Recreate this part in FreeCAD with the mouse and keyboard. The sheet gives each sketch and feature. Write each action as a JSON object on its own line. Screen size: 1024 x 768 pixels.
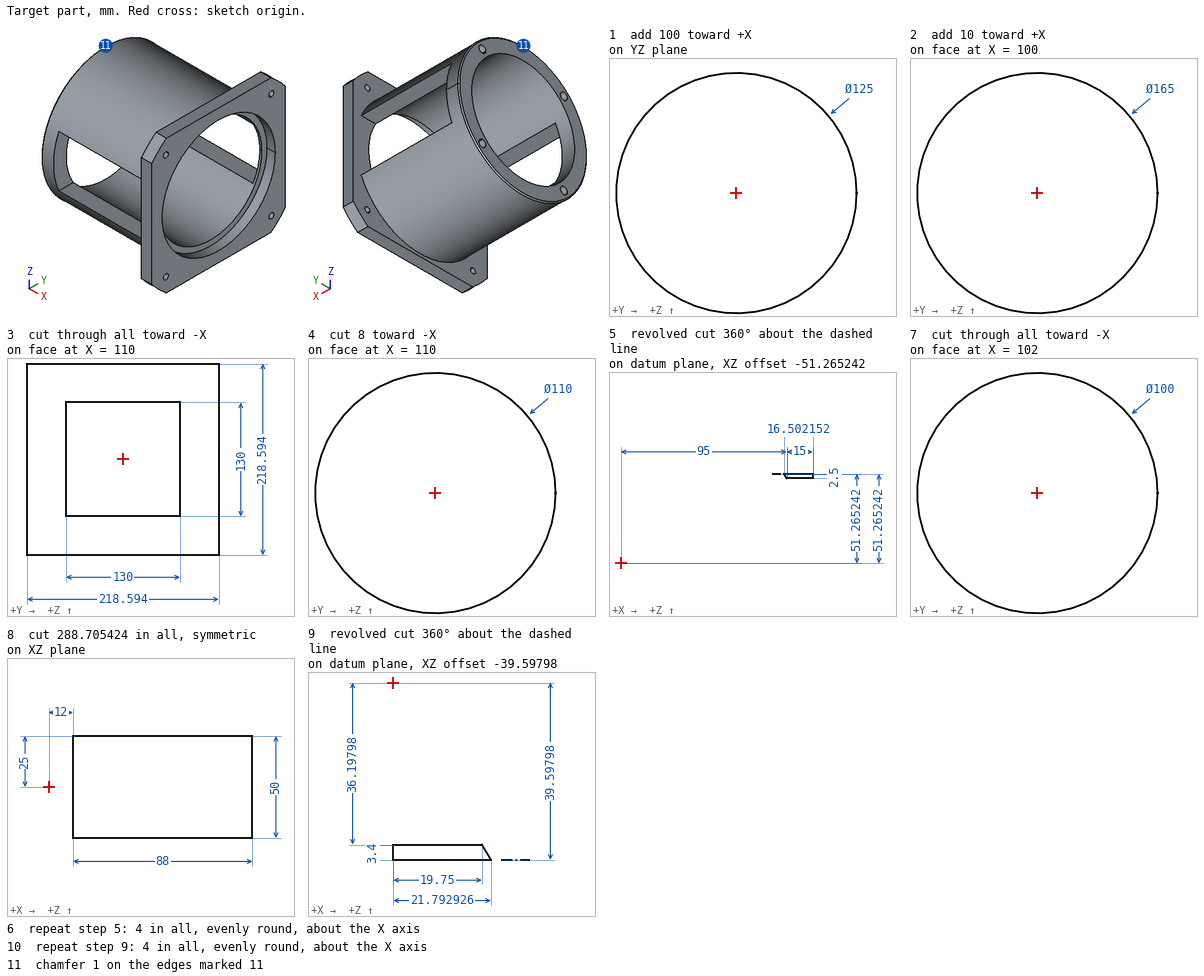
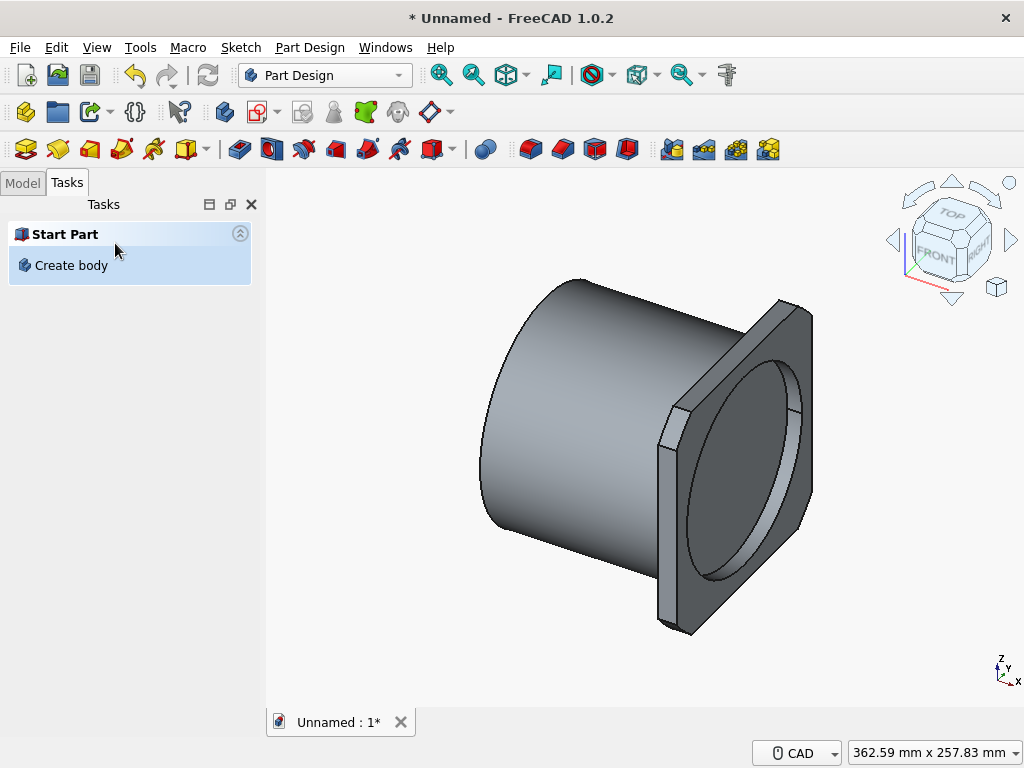
{"action": "left_click", "coordinate": [23, 182]}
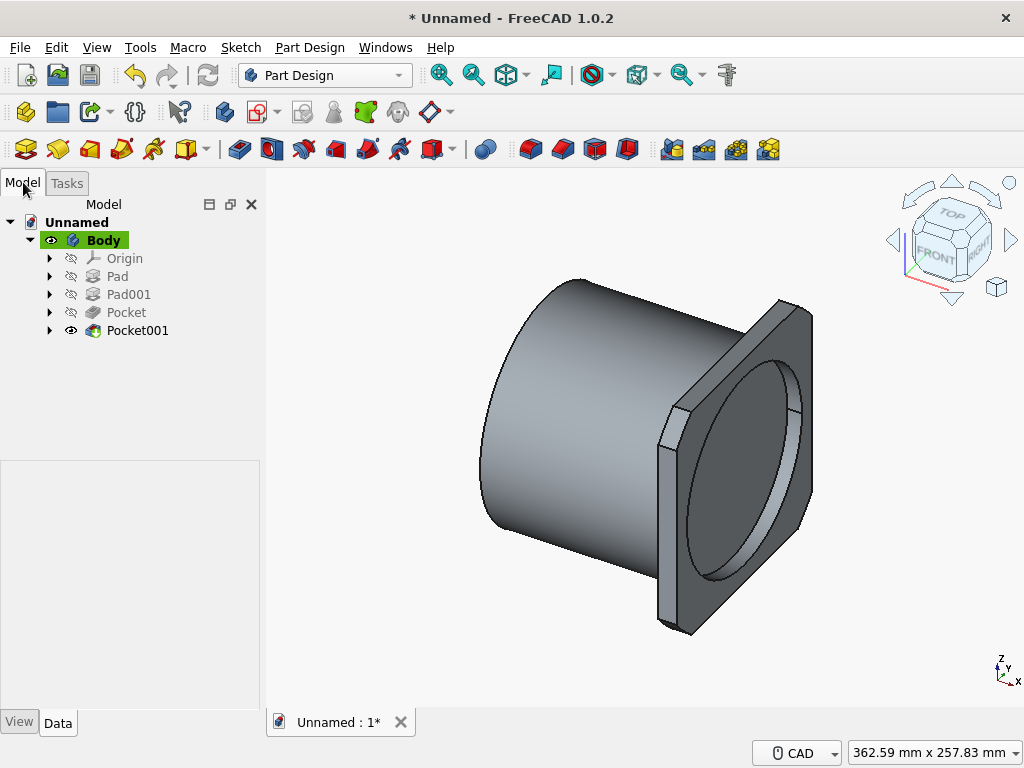
{"action": "left_click", "coordinate": [50, 258]}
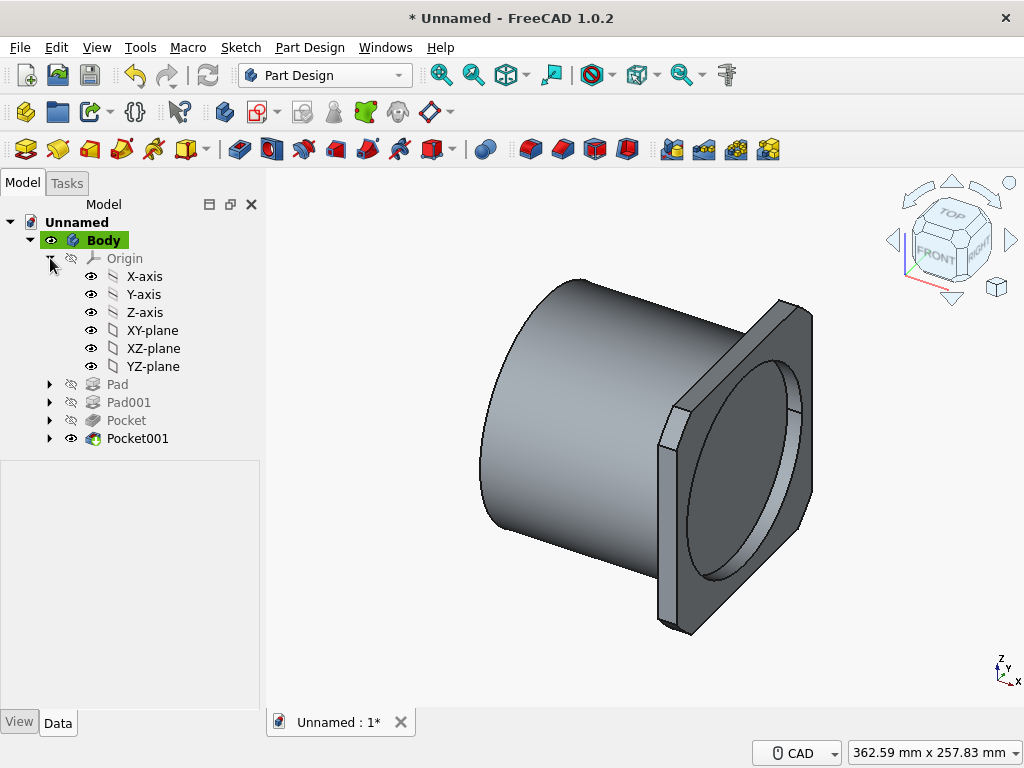
{"action": "left_click", "coordinate": [136, 348]}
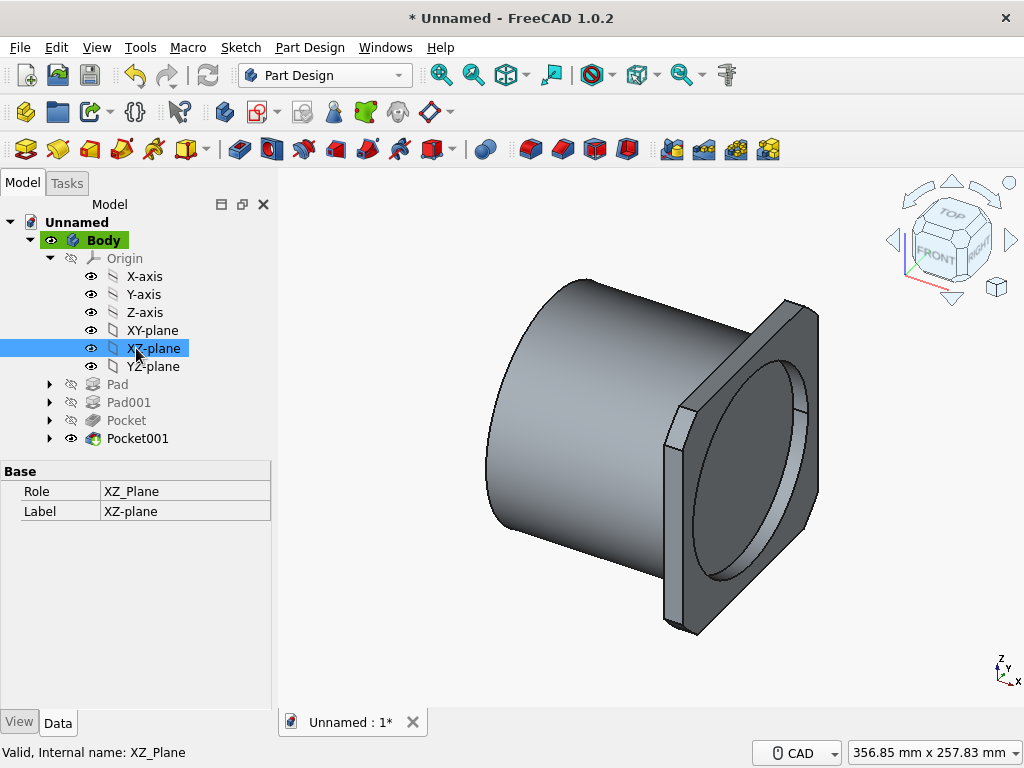
{"action": "left_click", "coordinate": [430, 112]}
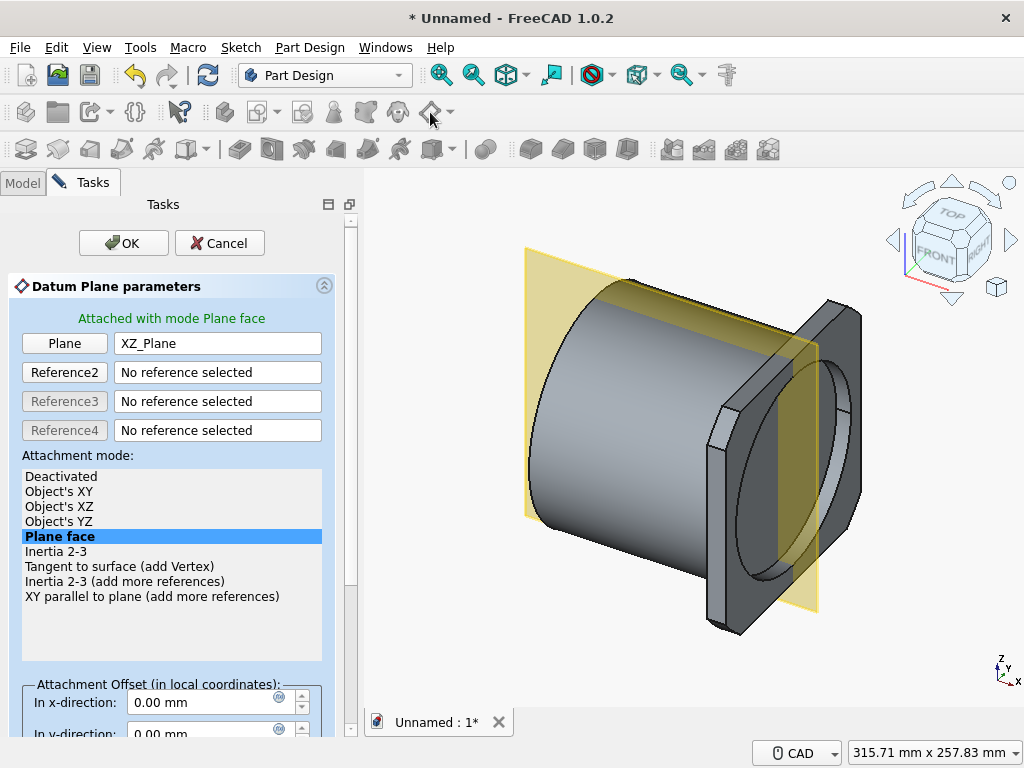
{"action": "scroll", "coordinate": [351, 475], "scroll_direction": "down", "scroll_amount": 2}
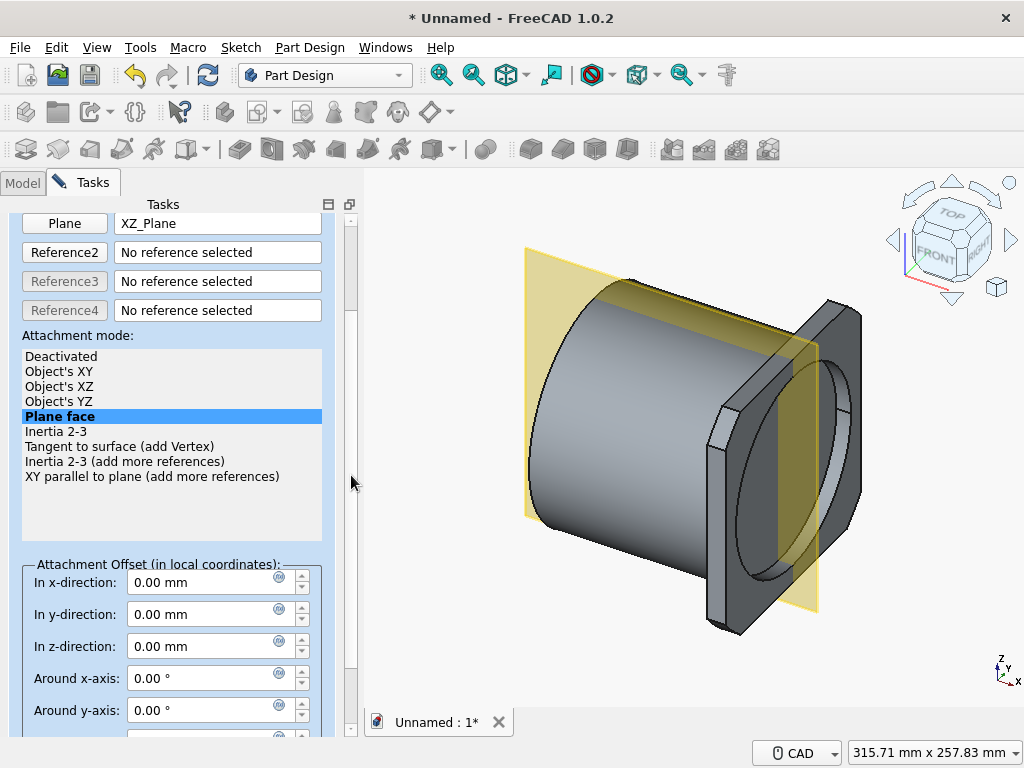
{"action": "triple_click", "coordinate": [210, 646]}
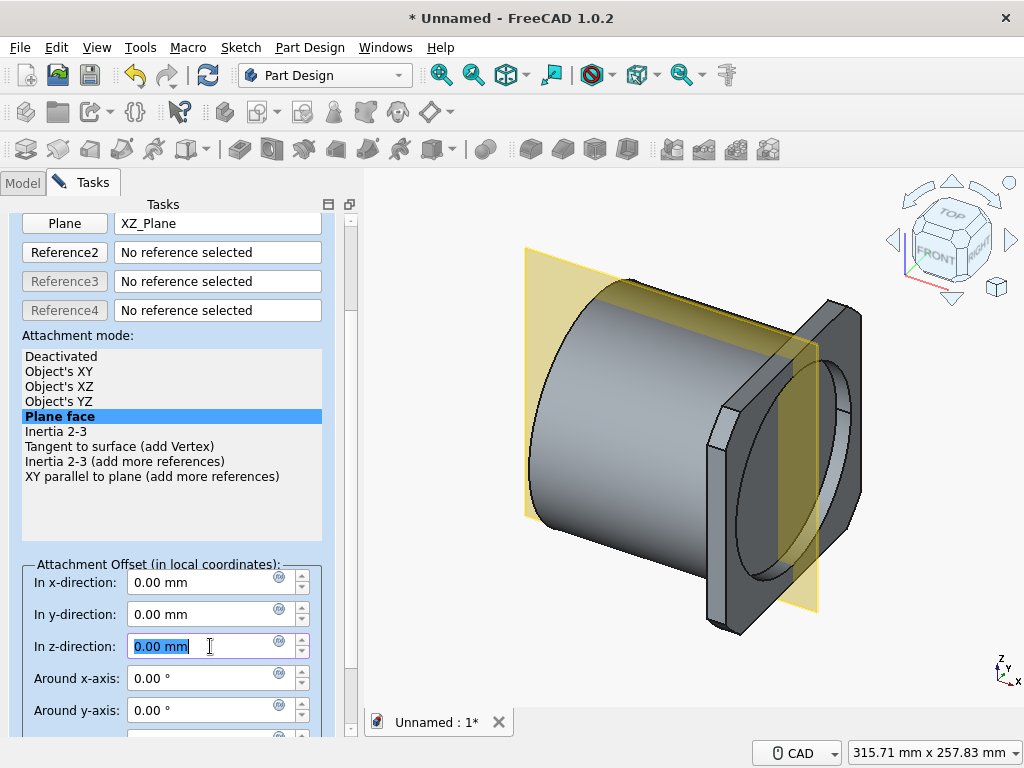
{"action": "type", "text": "-51.265242"}
{"action": "key", "text": "Tab"}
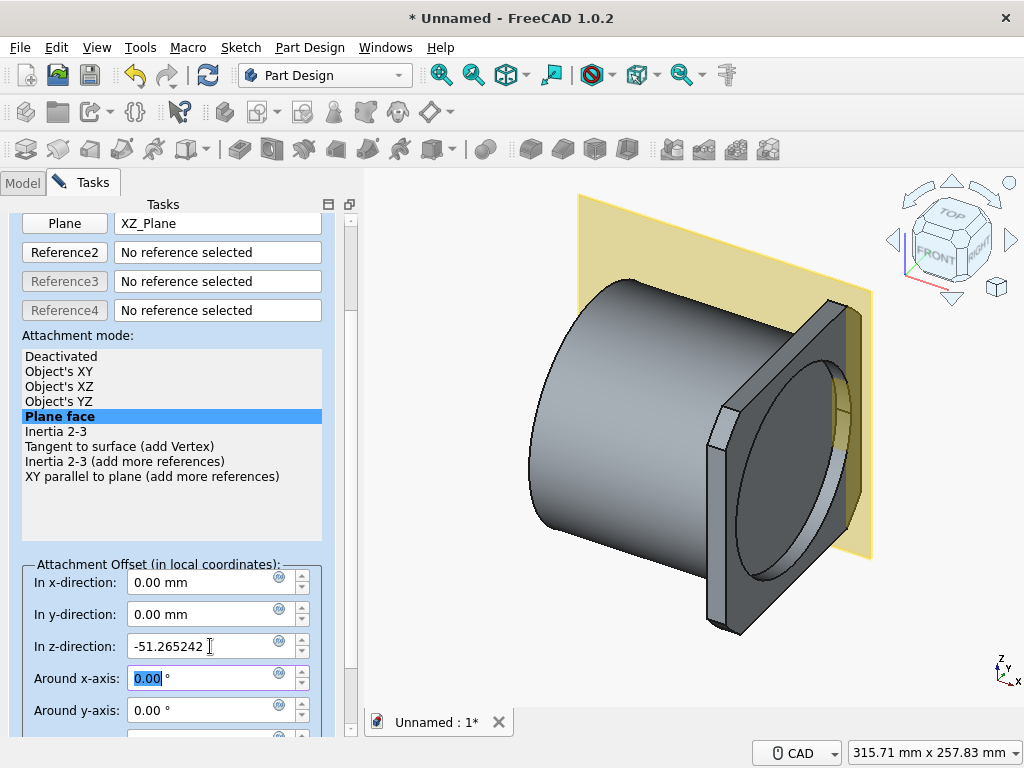
{"action": "scroll", "coordinate": [351, 475], "scroll_direction": "up", "scroll_amount": 3}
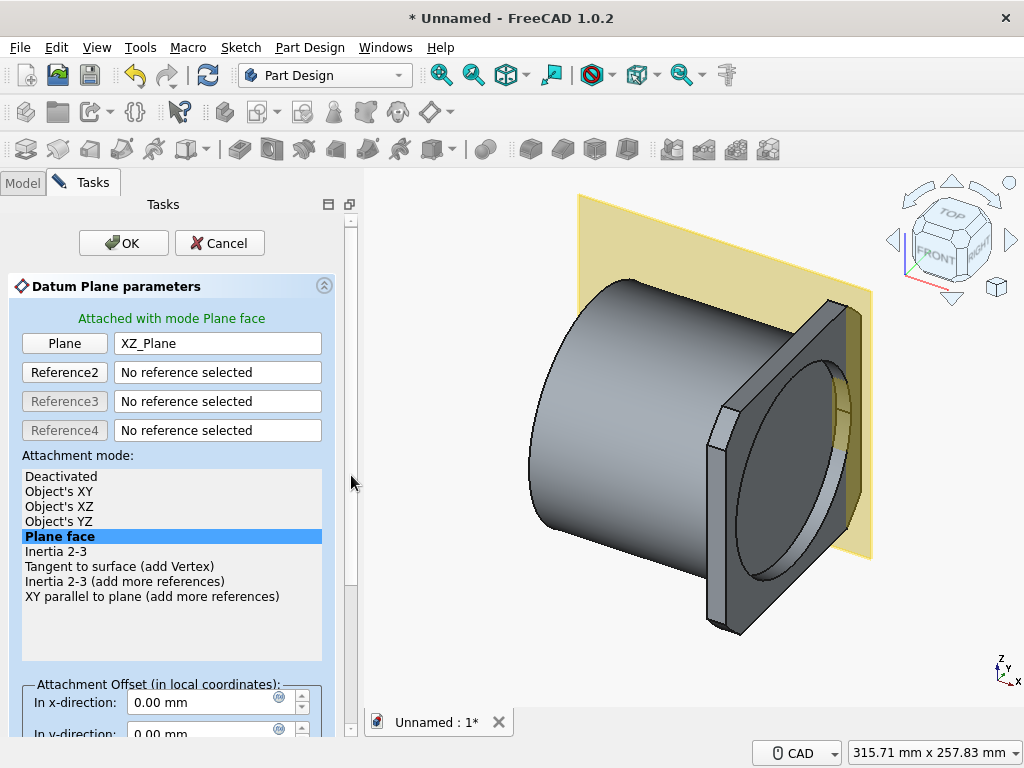
{"action": "left_click", "coordinate": [124, 243]}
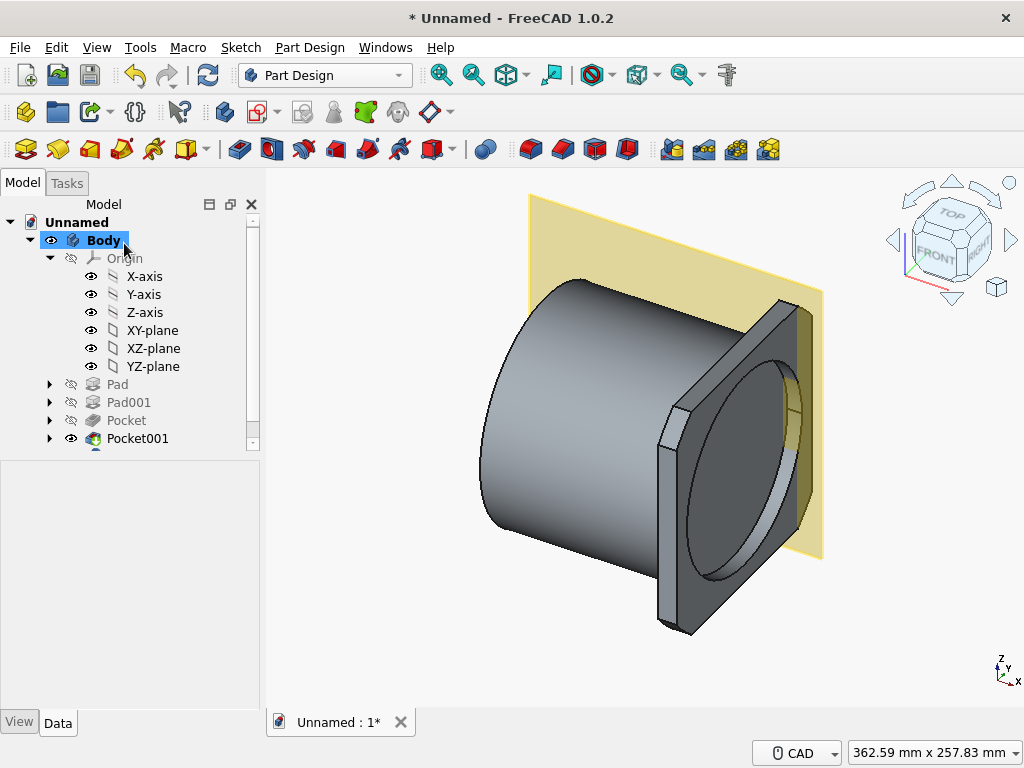
{"action": "scroll", "coordinate": [100, 326], "scroll_direction": "down", "scroll_amount": 3}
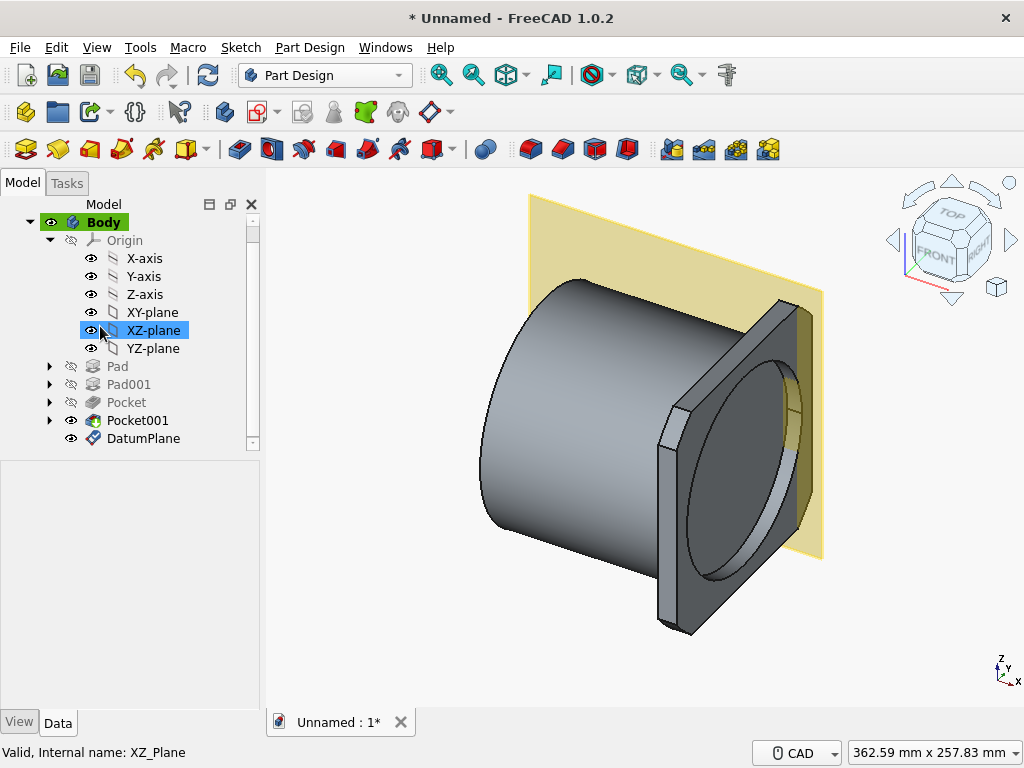
{"action": "left_click", "coordinate": [116, 438]}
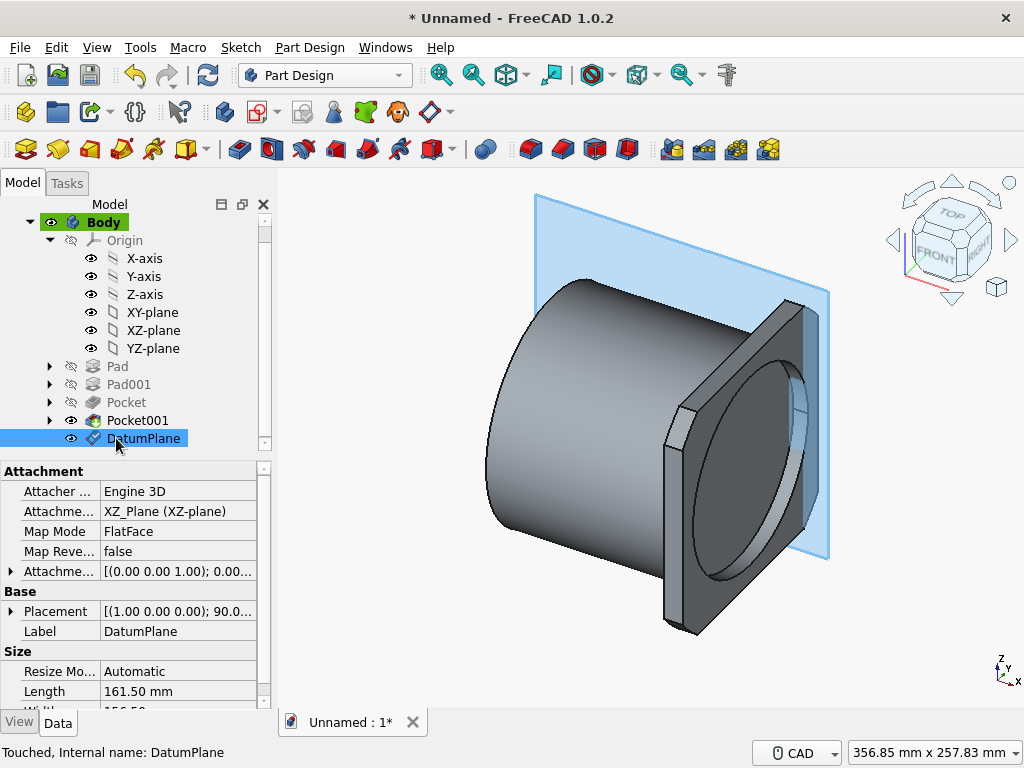
{"action": "left_click", "coordinate": [258, 112]}